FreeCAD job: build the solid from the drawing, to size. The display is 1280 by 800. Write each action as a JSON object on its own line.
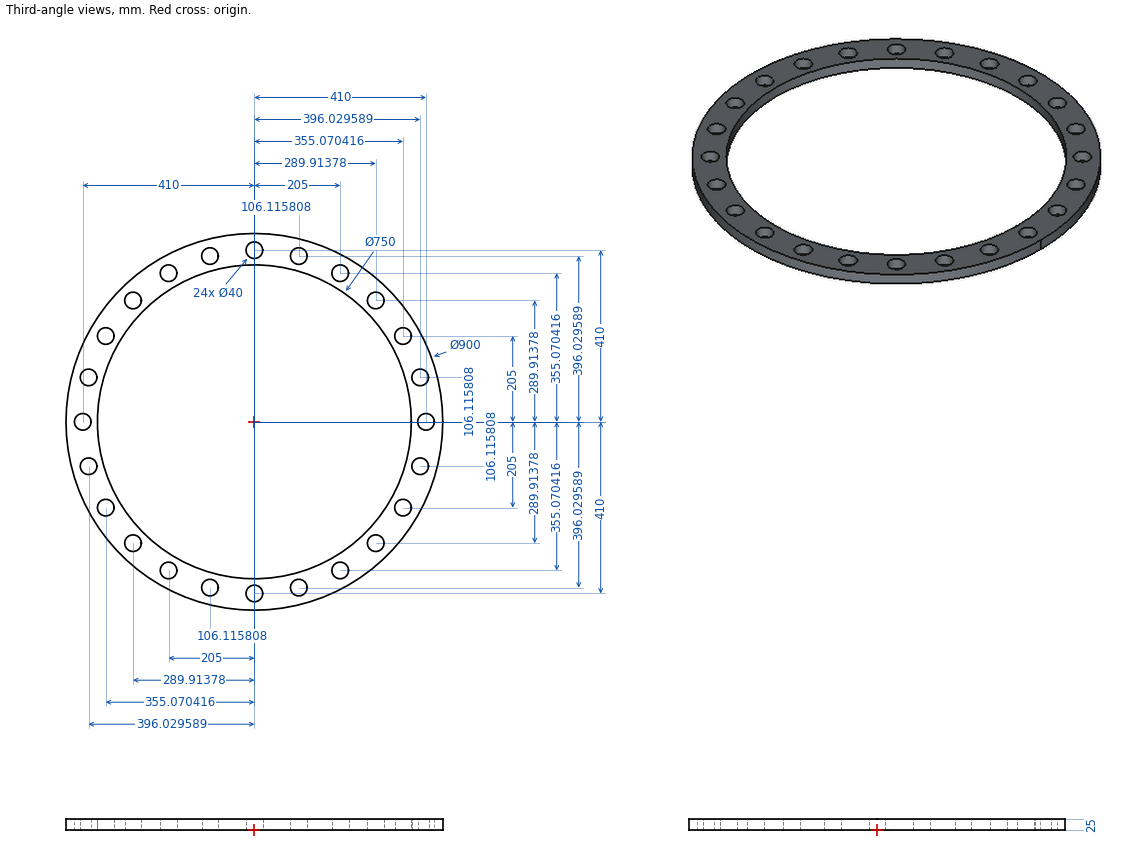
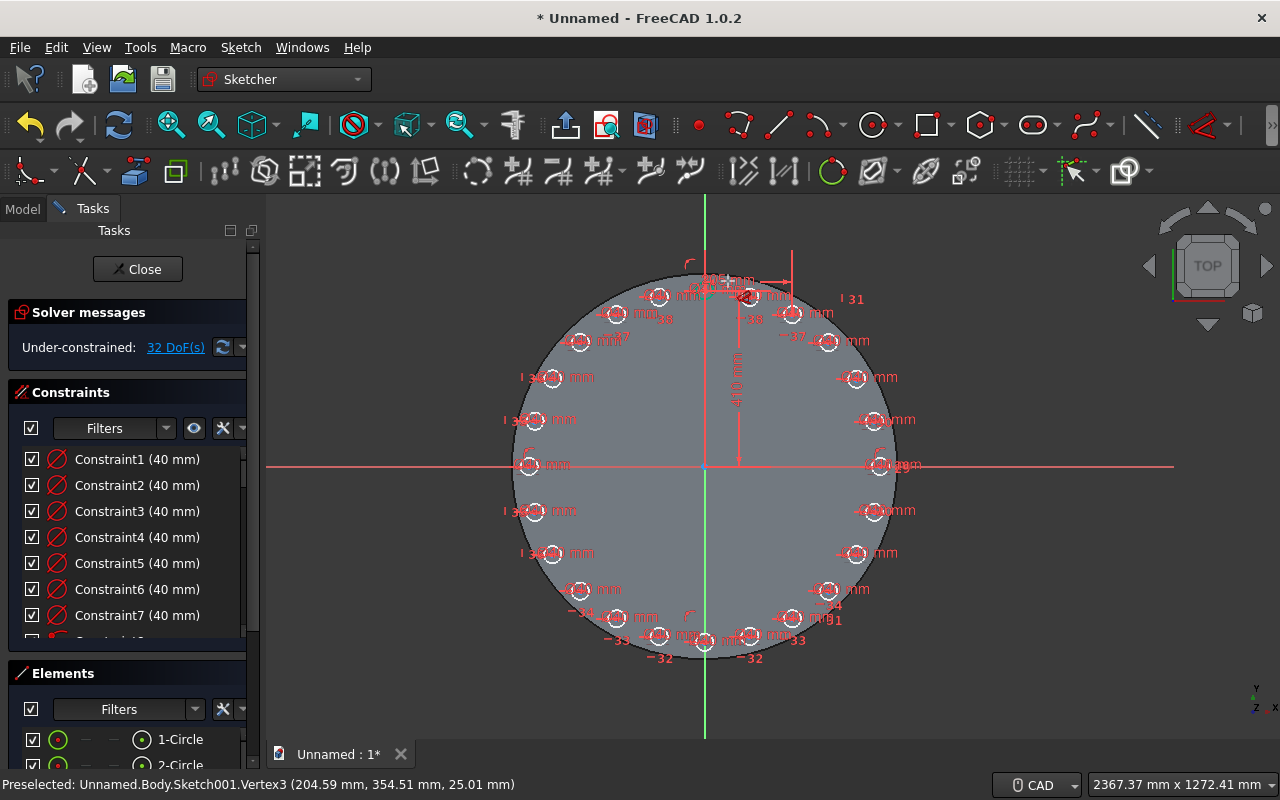
{"action": "left_click", "coordinate": [857, 379]}
{"action": "left_click", "coordinate": [891, 403]}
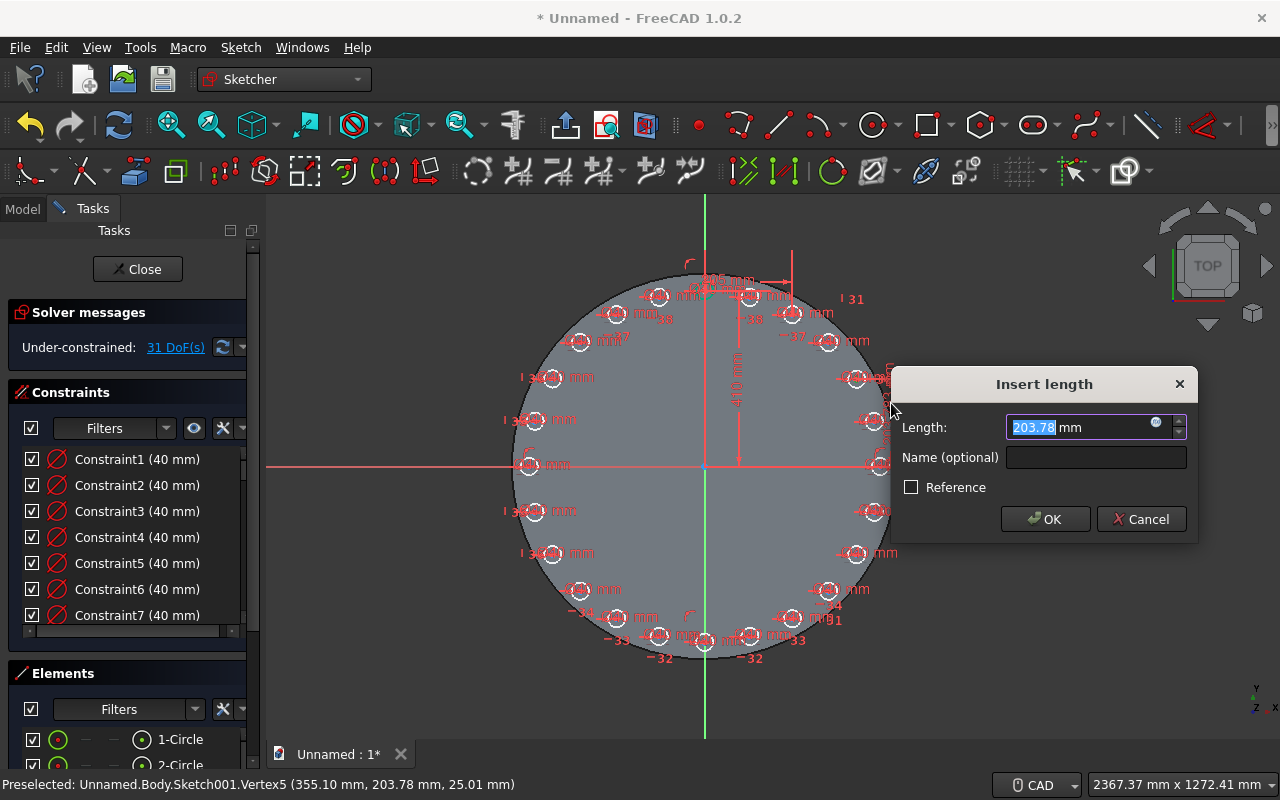
{"action": "type", "text": "205"}
{"action": "key", "text": "Return"}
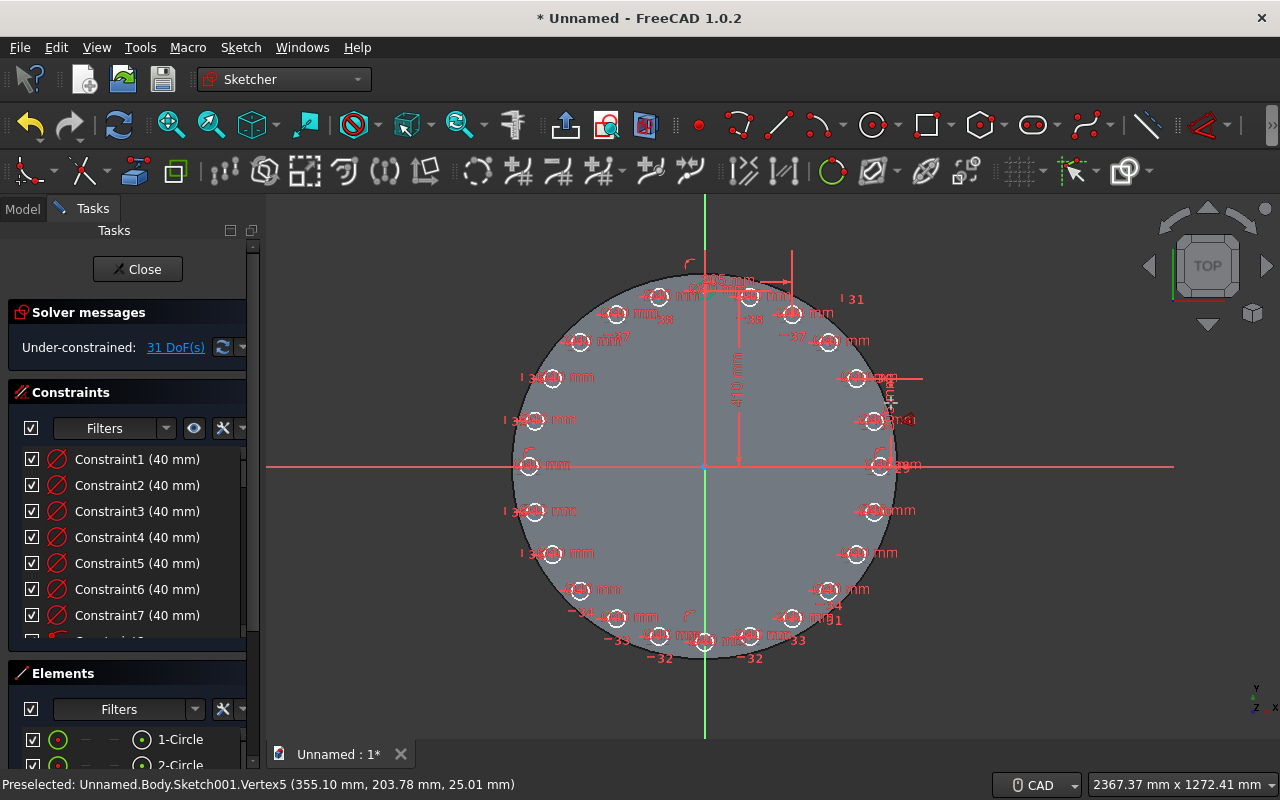
{"action": "left_click", "coordinate": [880, 467]}
{"action": "left_click", "coordinate": [792, 501]}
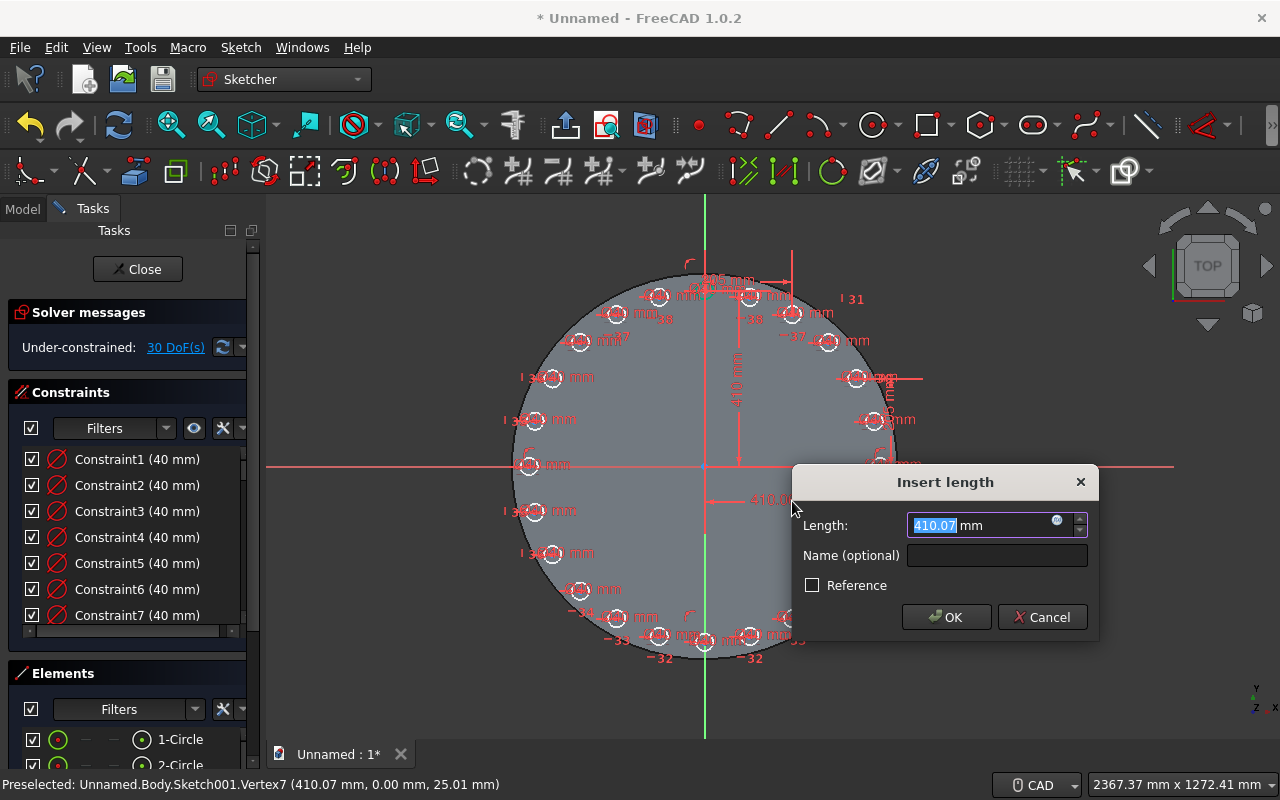
{"action": "type", "text": "410"}
{"action": "key", "text": "Return"}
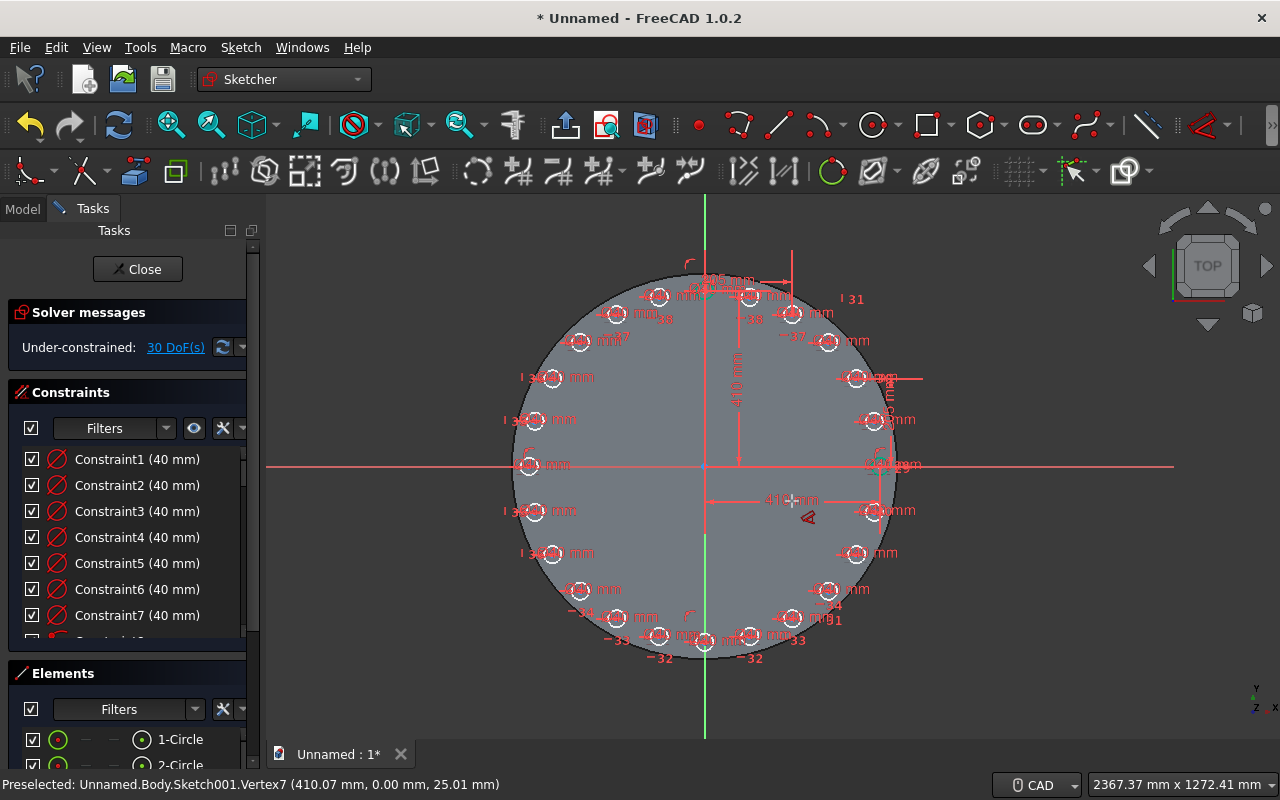
{"action": "left_click", "coordinate": [857, 555]}
{"action": "left_click", "coordinate": [891, 490]}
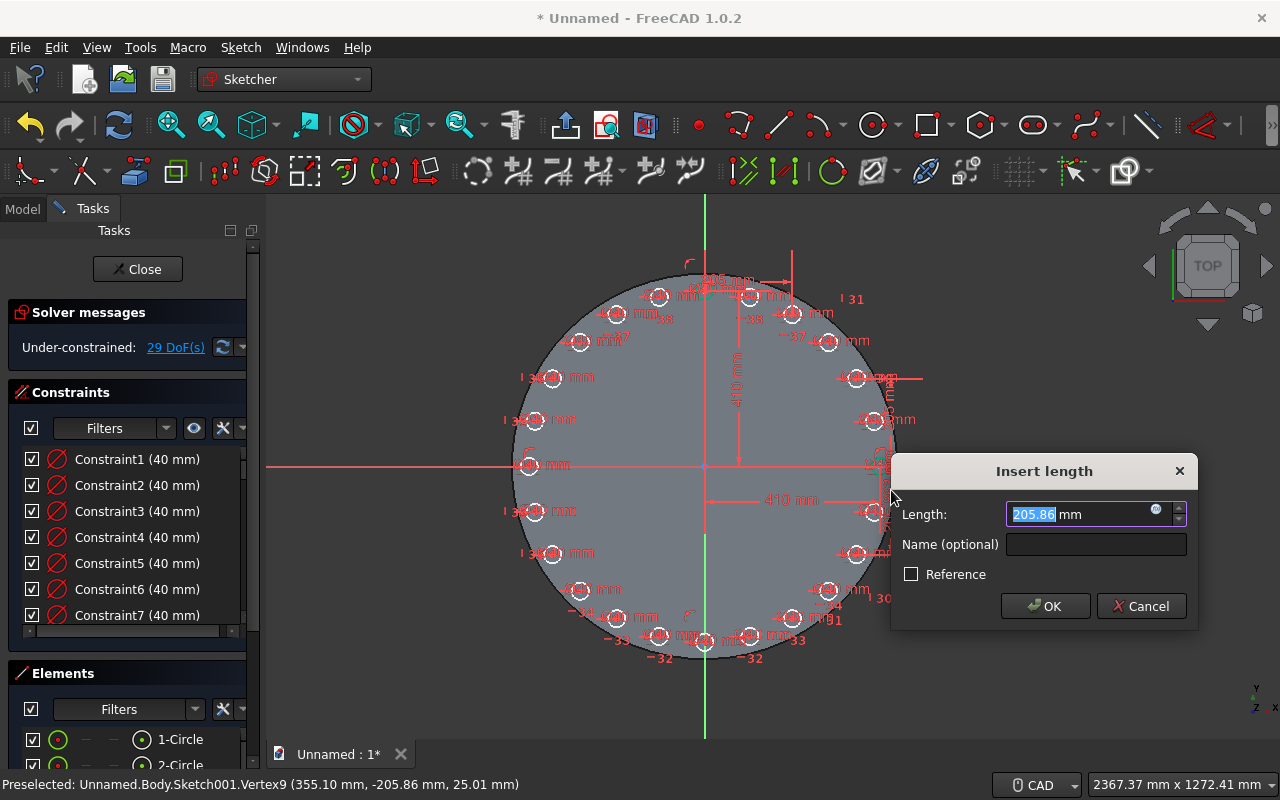
{"action": "type", "text": "205"}
{"action": "key", "text": "Return"}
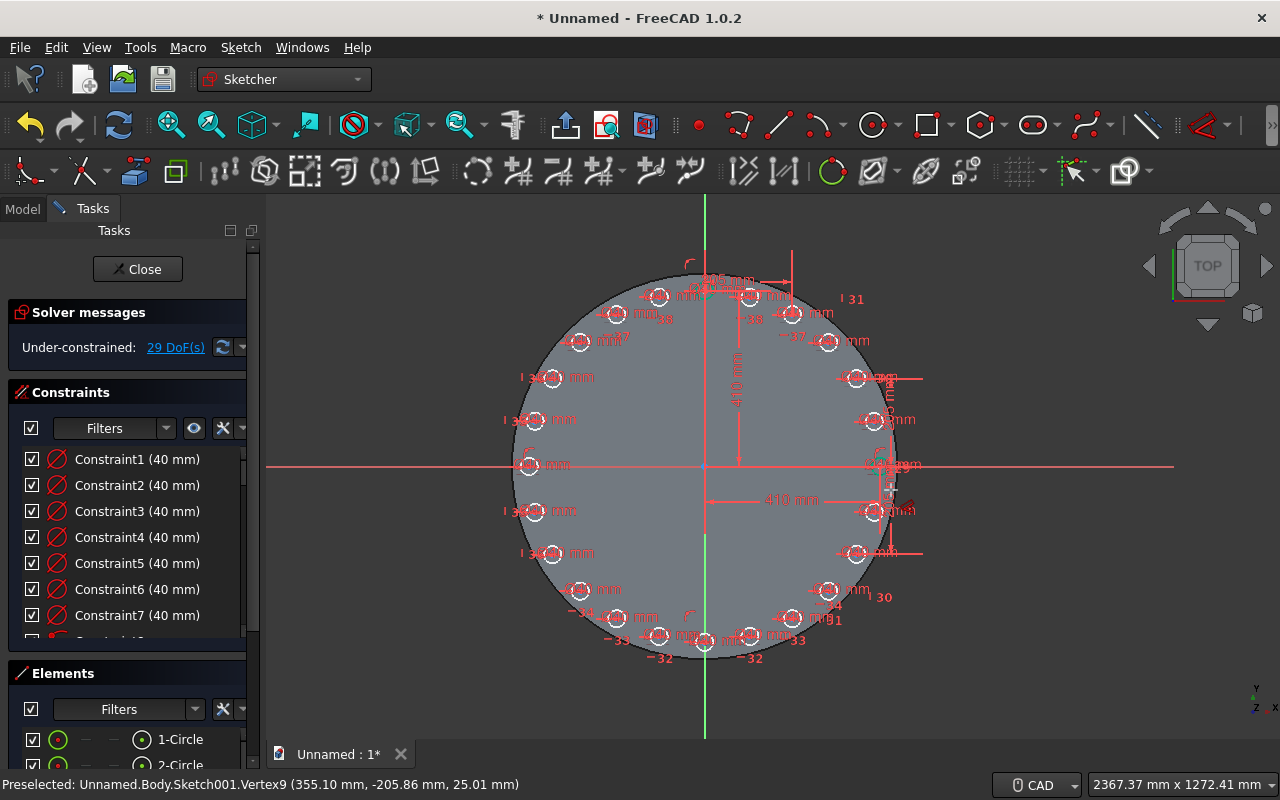
{"action": "left_click", "coordinate": [792, 619]}
{"action": "left_click", "coordinate": [728, 653]}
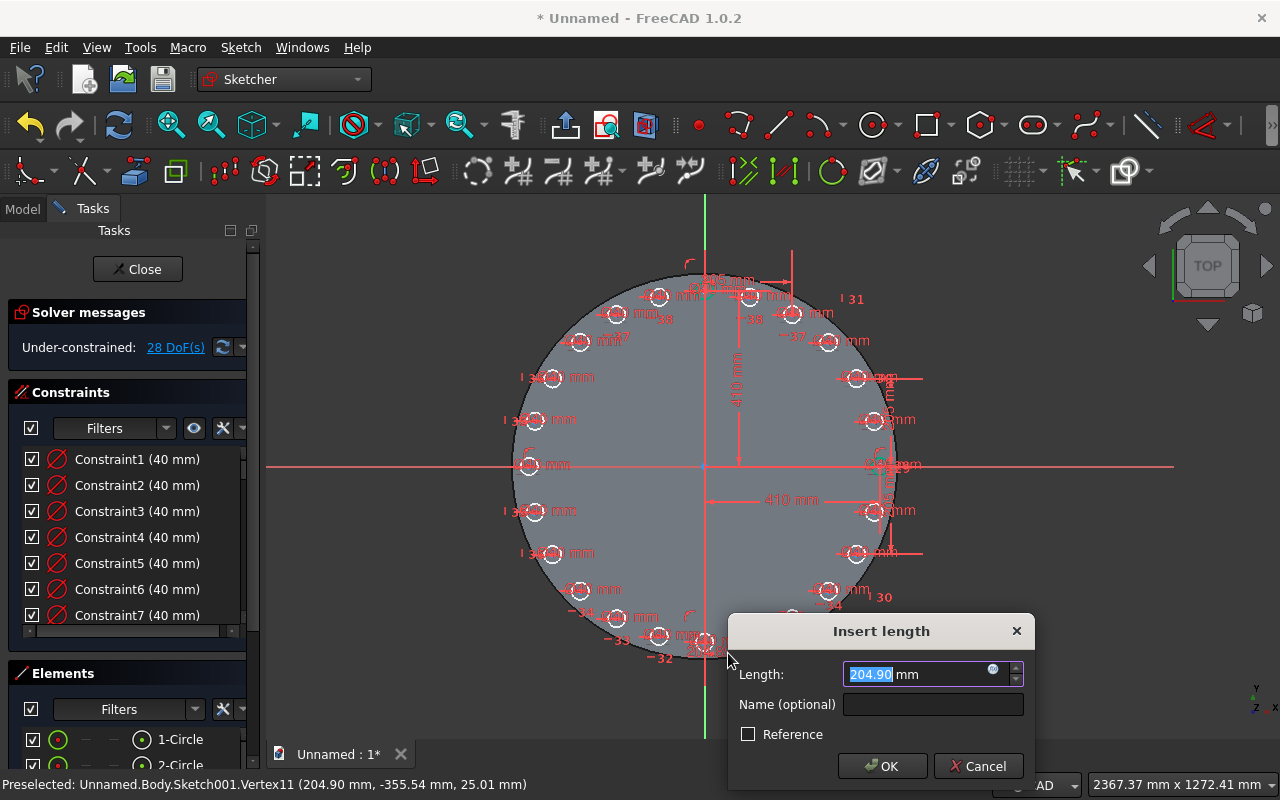
{"action": "type", "text": "205"}
{"action": "key", "text": "Return"}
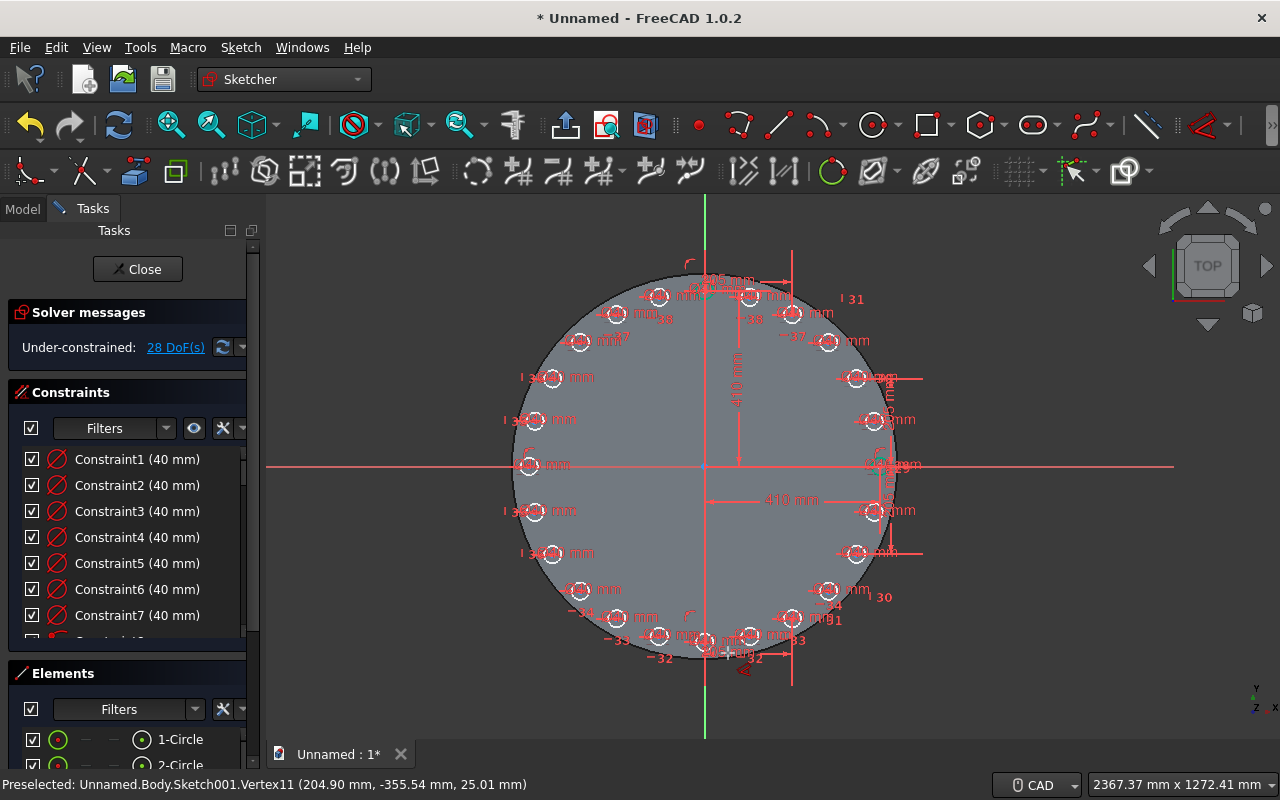
{"action": "left_click", "coordinate": [705, 642]}
{"action": "left_click", "coordinate": [739, 554]}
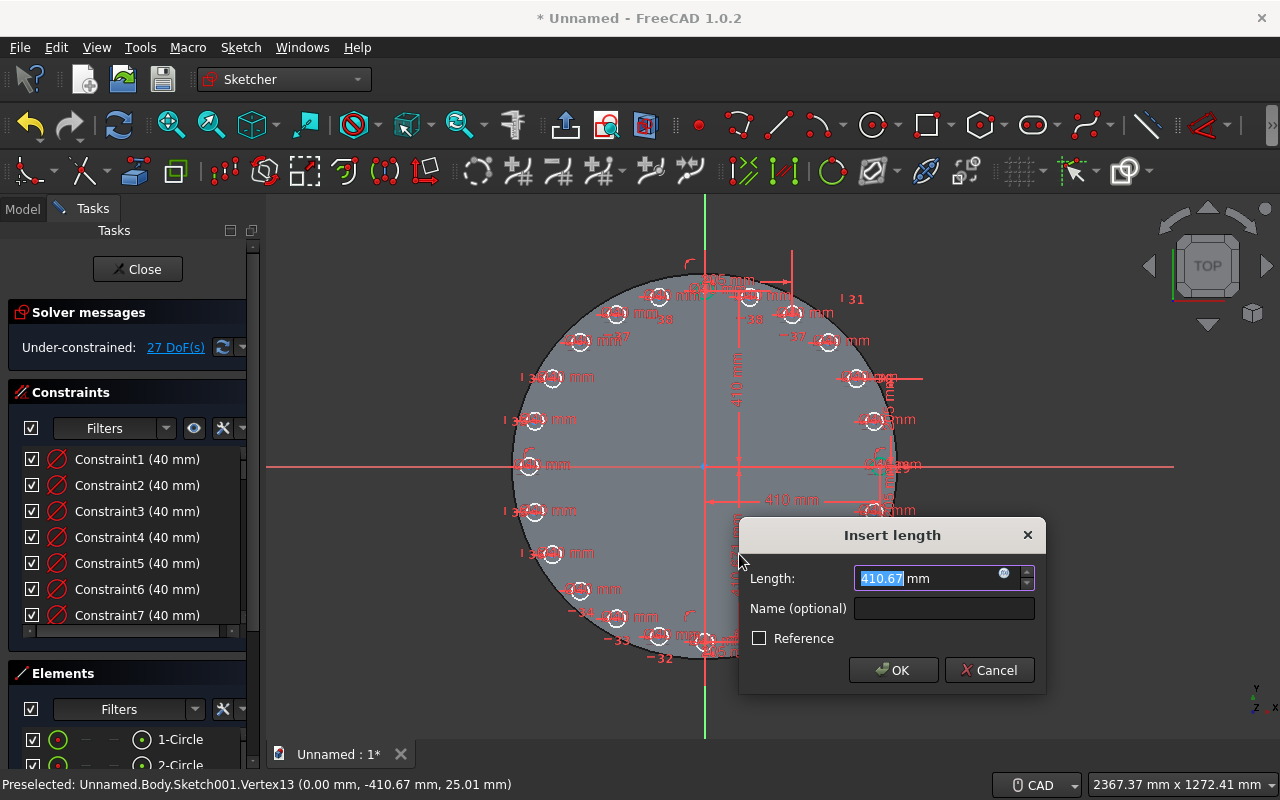
{"action": "type", "text": "410"}
{"action": "key", "text": "Return"}